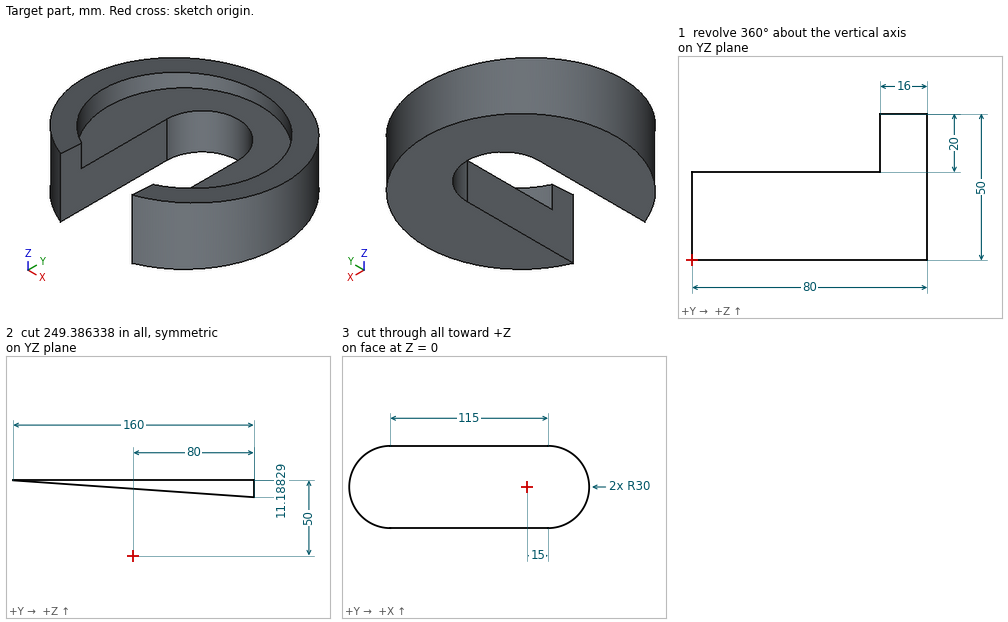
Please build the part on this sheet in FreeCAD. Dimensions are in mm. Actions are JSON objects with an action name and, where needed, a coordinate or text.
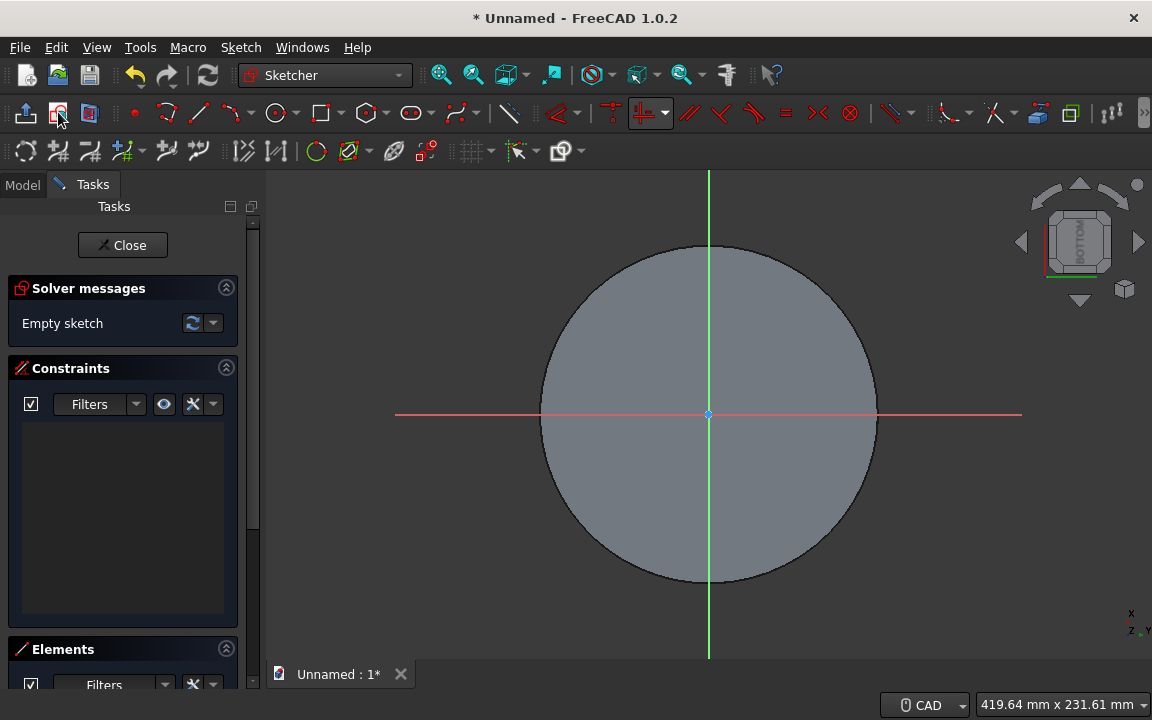
{"action": "left_click", "coordinate": [412, 114]}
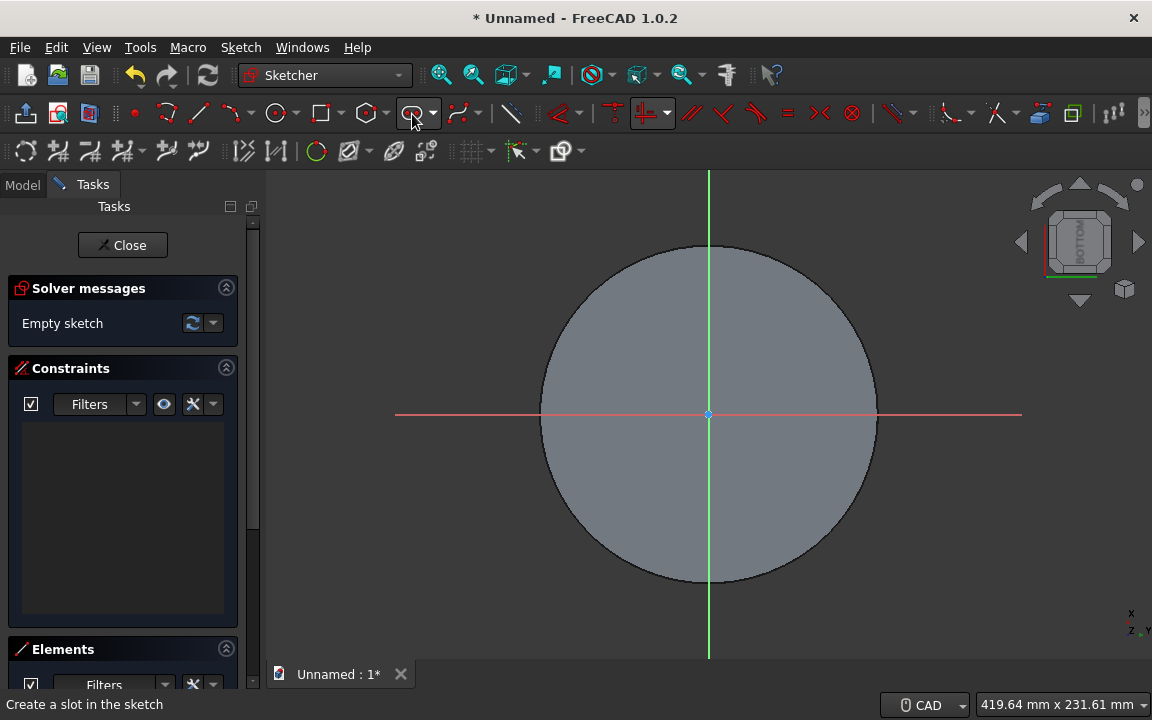
{"action": "left_click", "coordinate": [498, 415]}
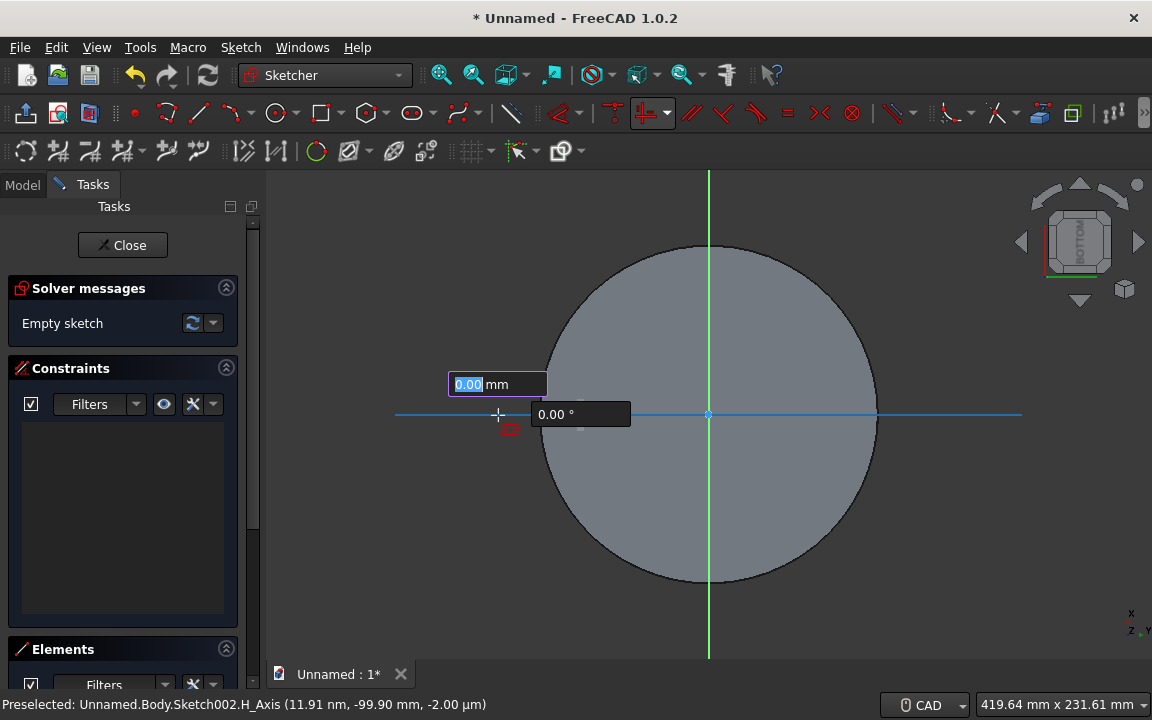
{"action": "left_click", "coordinate": [741, 406]}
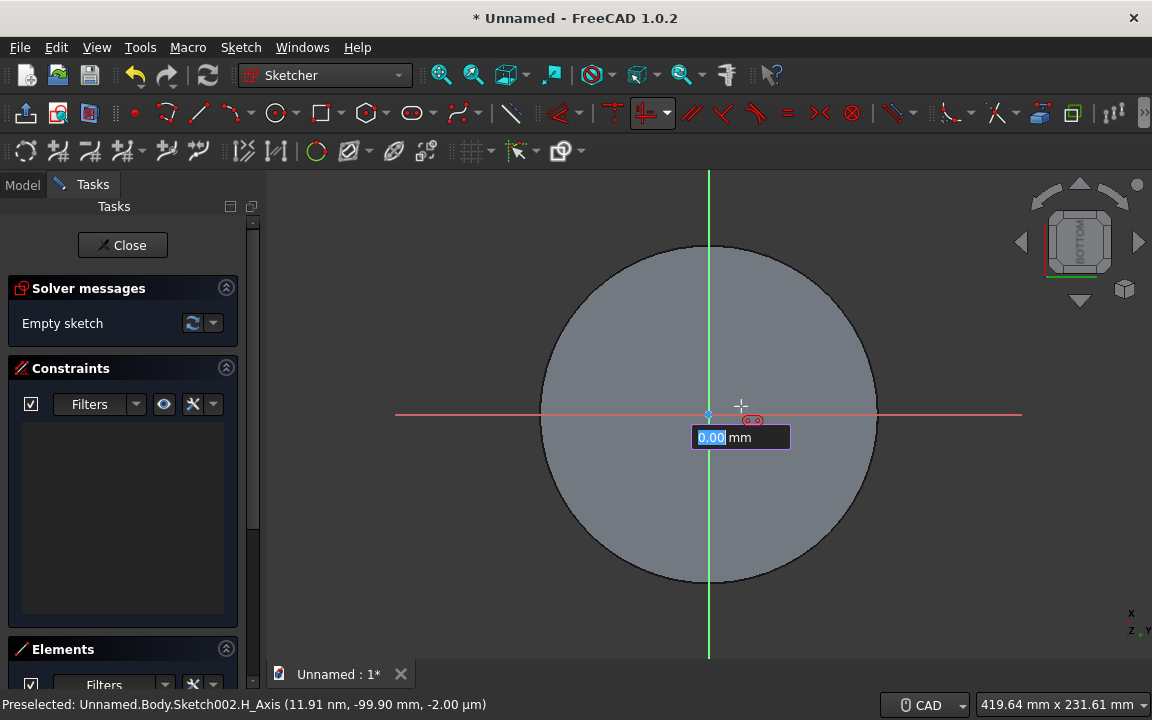
{"action": "left_click", "coordinate": [619, 351]}
{"action": "key", "text": "Escape"}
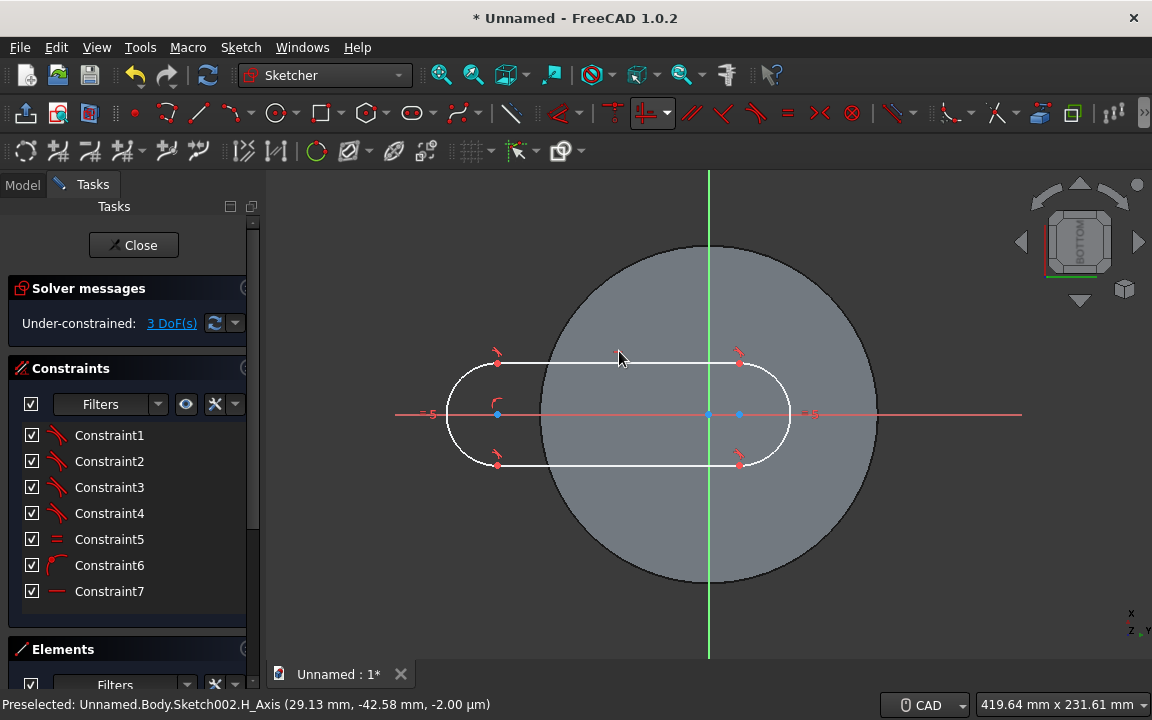
{"action": "left_click", "coordinate": [558, 114]}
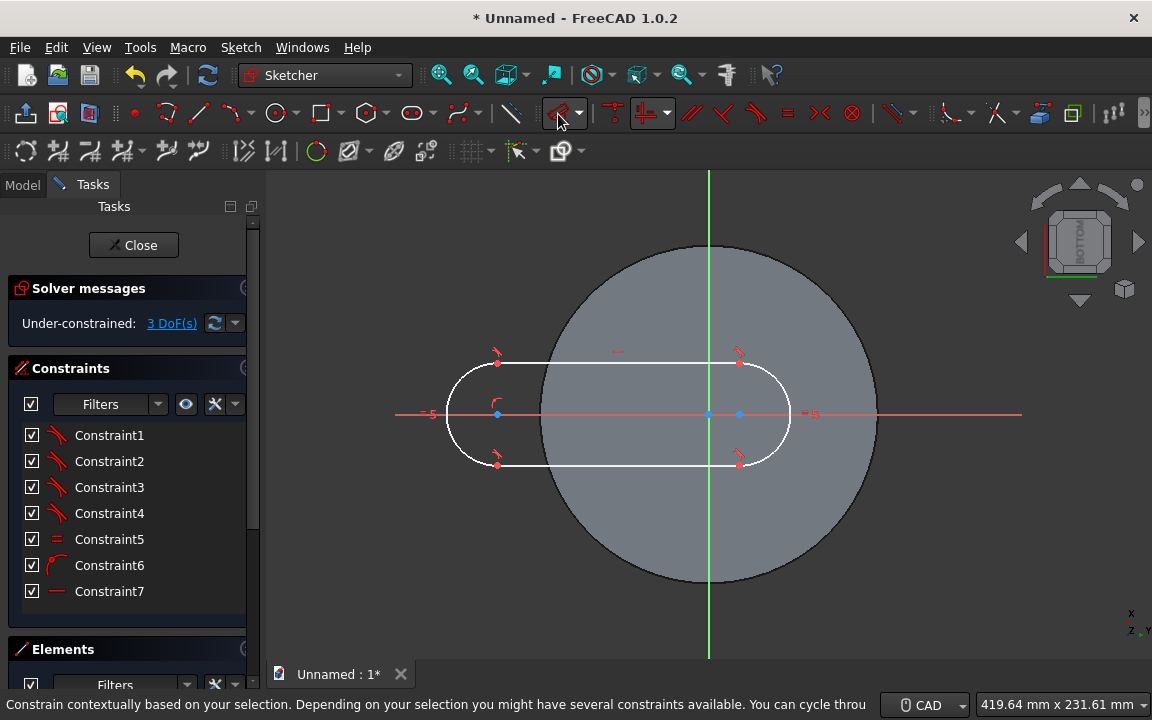
{"action": "left_click", "coordinate": [456, 384]}
{"action": "left_click", "coordinate": [430, 365]}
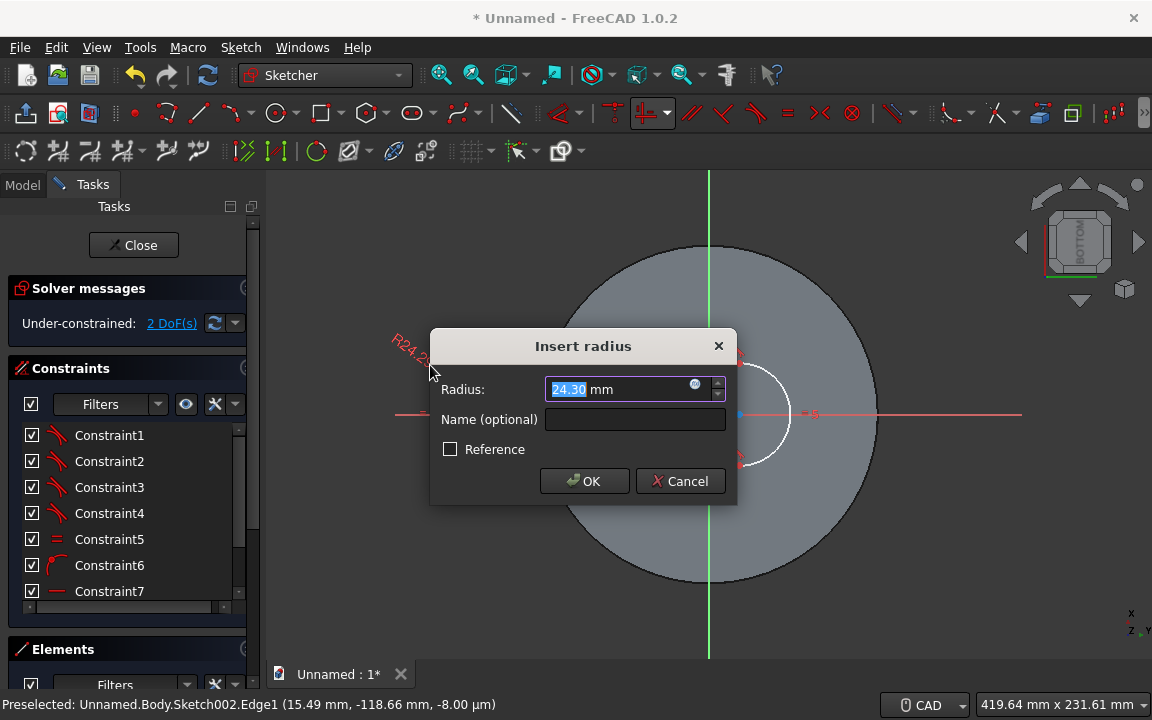
{"action": "type", "text": "30"}
{"action": "key", "text": "Return"}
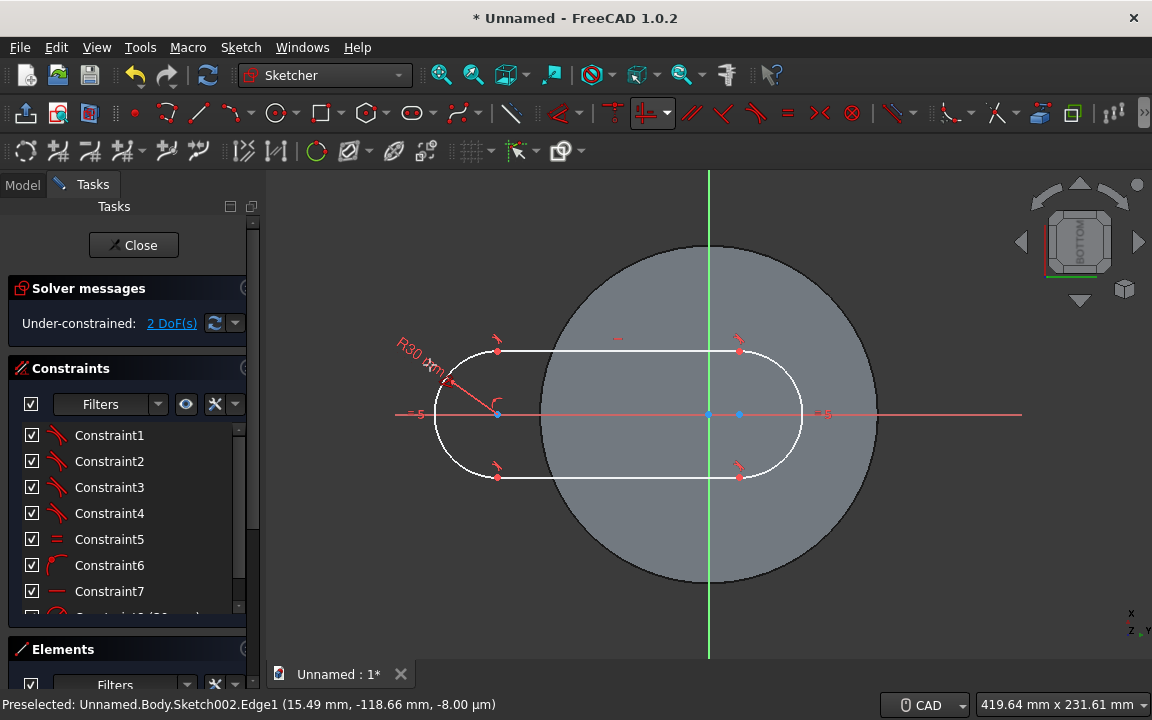
{"action": "left_click", "coordinate": [570, 351]}
{"action": "left_click", "coordinate": [619, 317]}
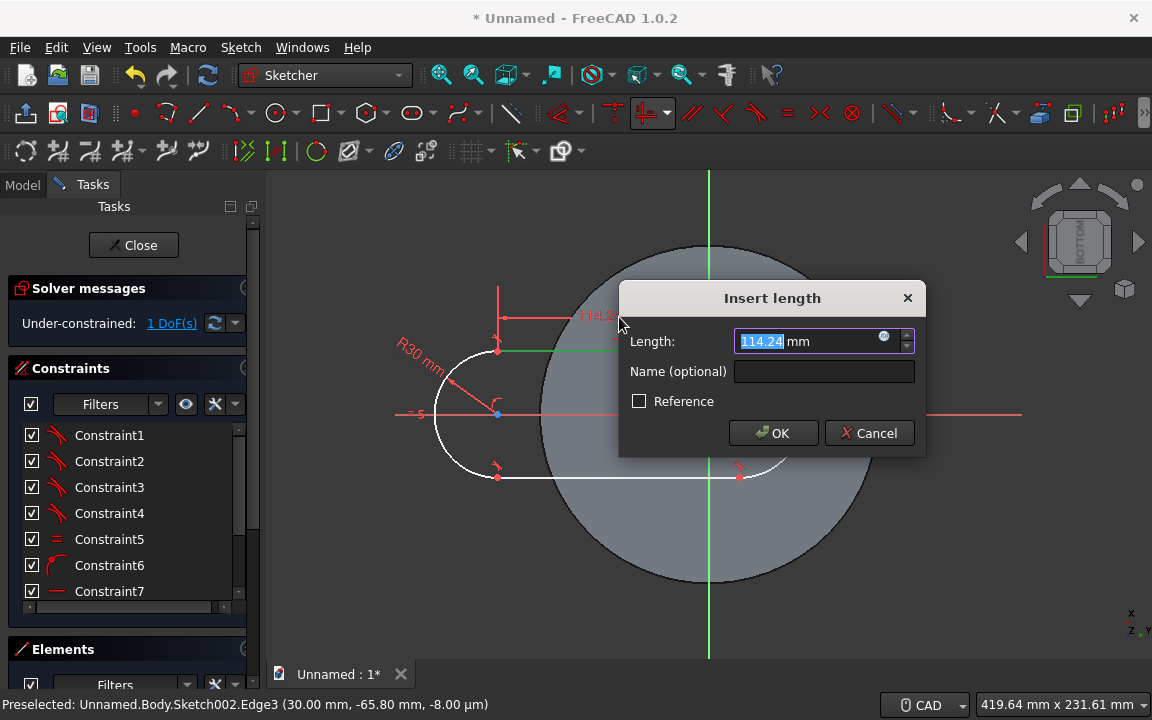
{"action": "type", "text": "115"}
{"action": "key", "text": "Return"}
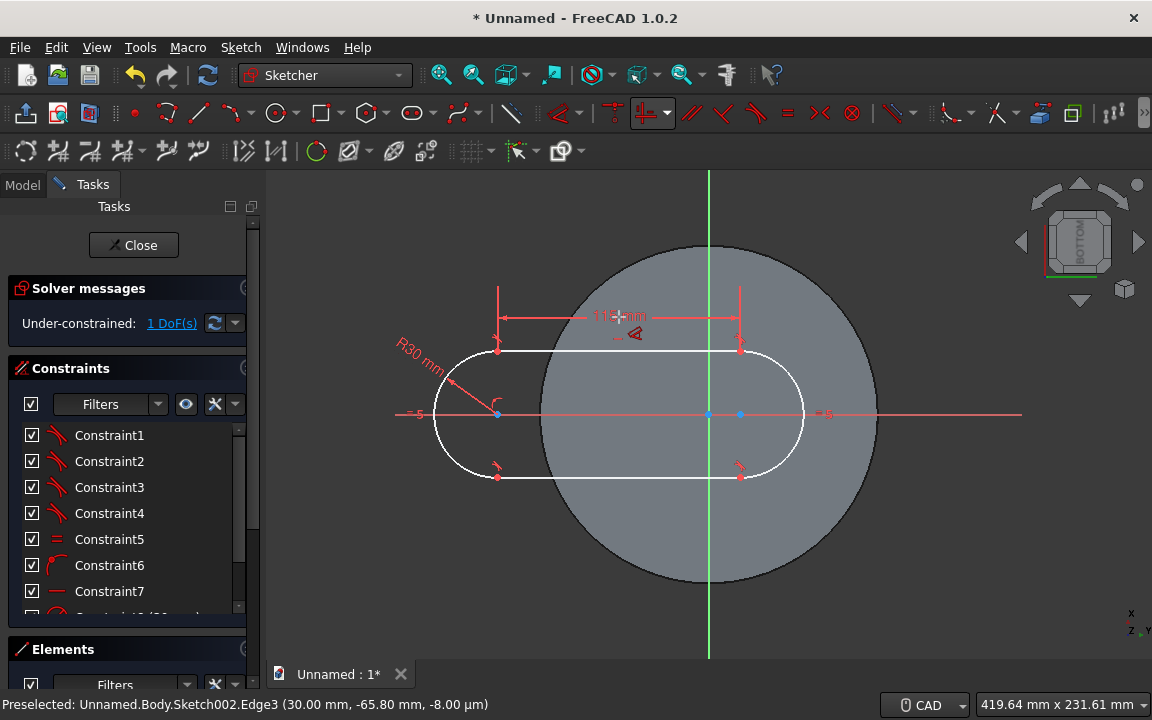
{"action": "scroll", "coordinate": [740, 478], "scroll_direction": "up", "scroll_amount": 2}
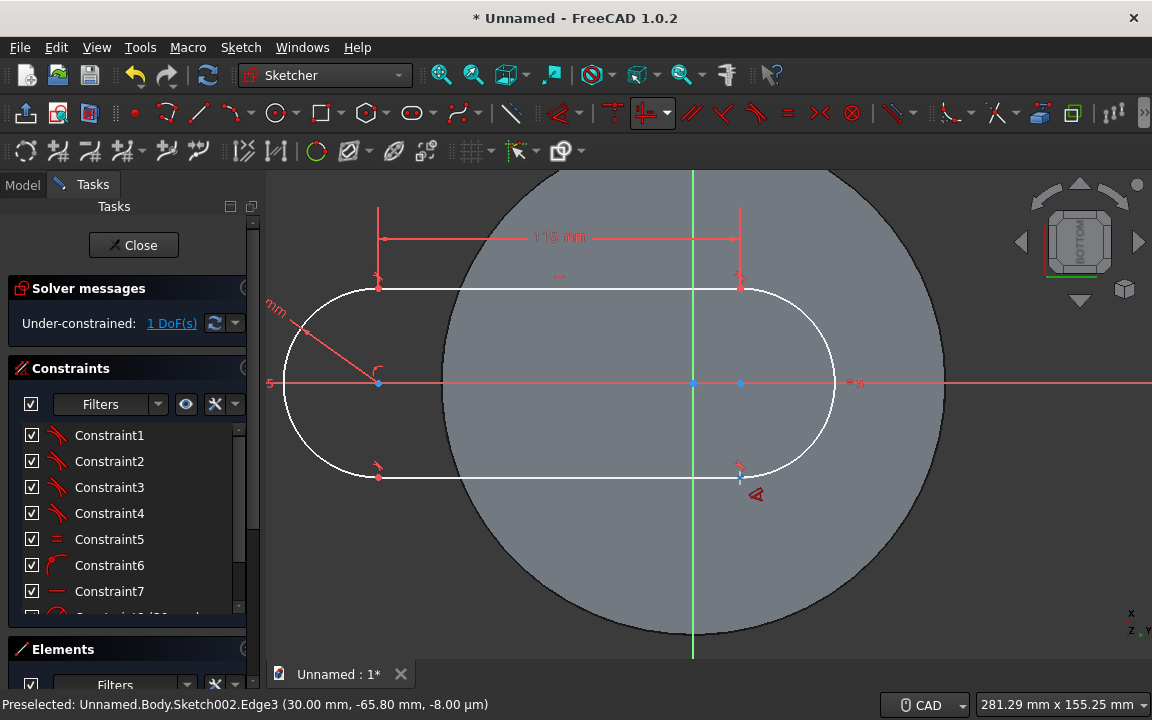
{"action": "left_click", "coordinate": [740, 477]}
{"action": "left_click", "coordinate": [717, 511]}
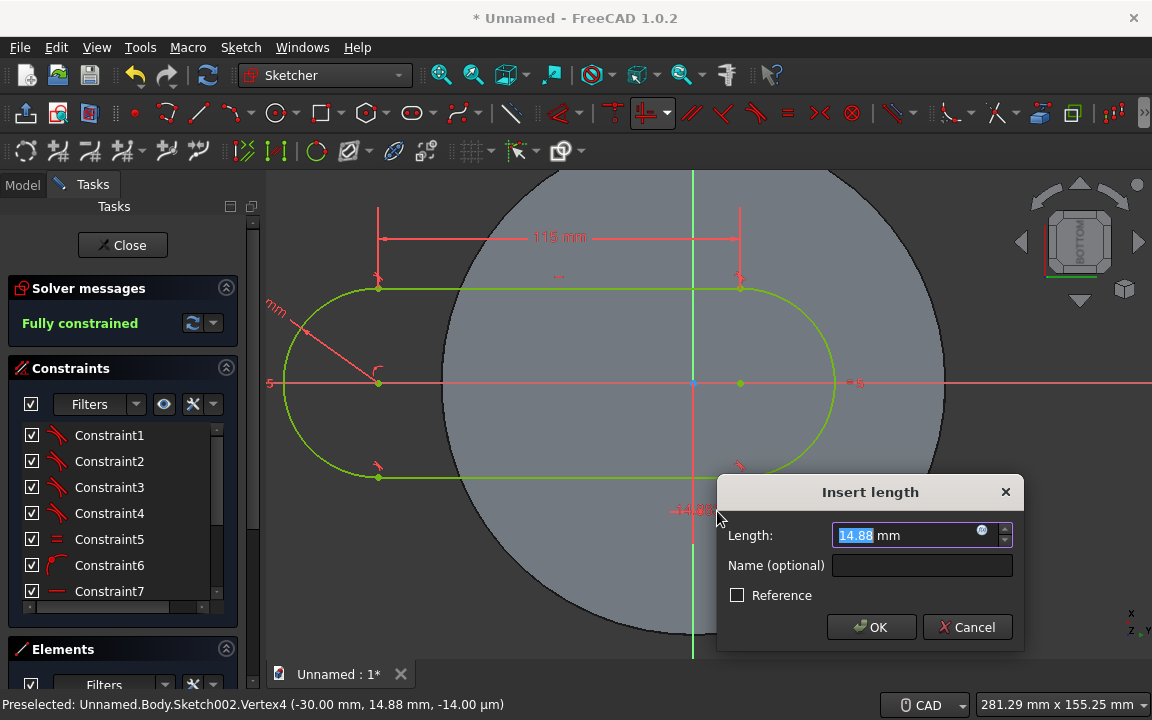
{"action": "type", "text": "15"}
{"action": "key", "text": "Return"}
{"action": "key", "text": "Escape"}